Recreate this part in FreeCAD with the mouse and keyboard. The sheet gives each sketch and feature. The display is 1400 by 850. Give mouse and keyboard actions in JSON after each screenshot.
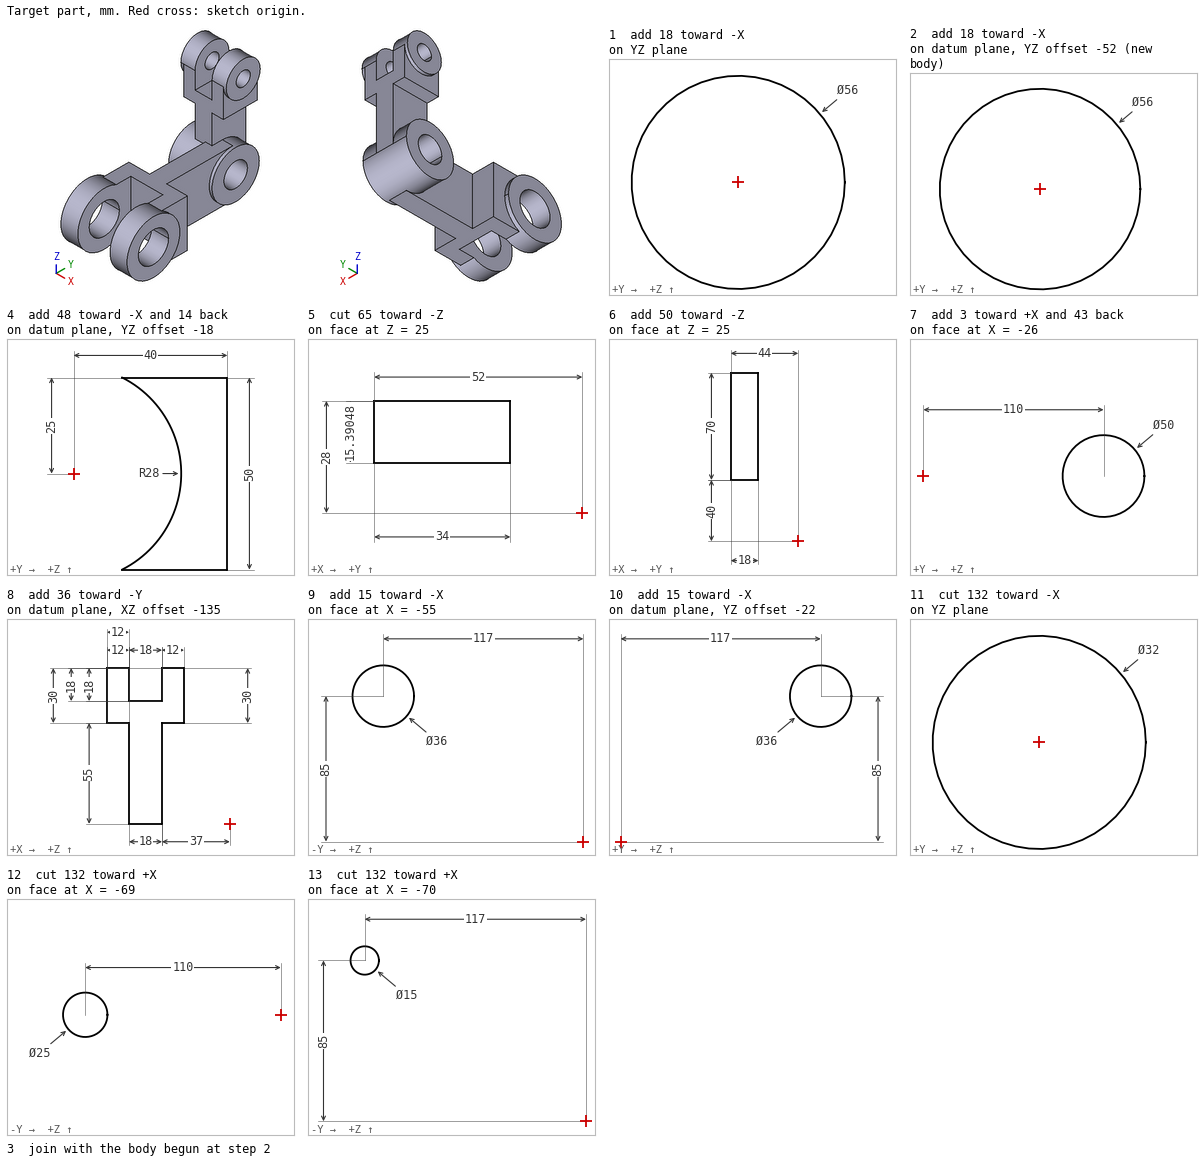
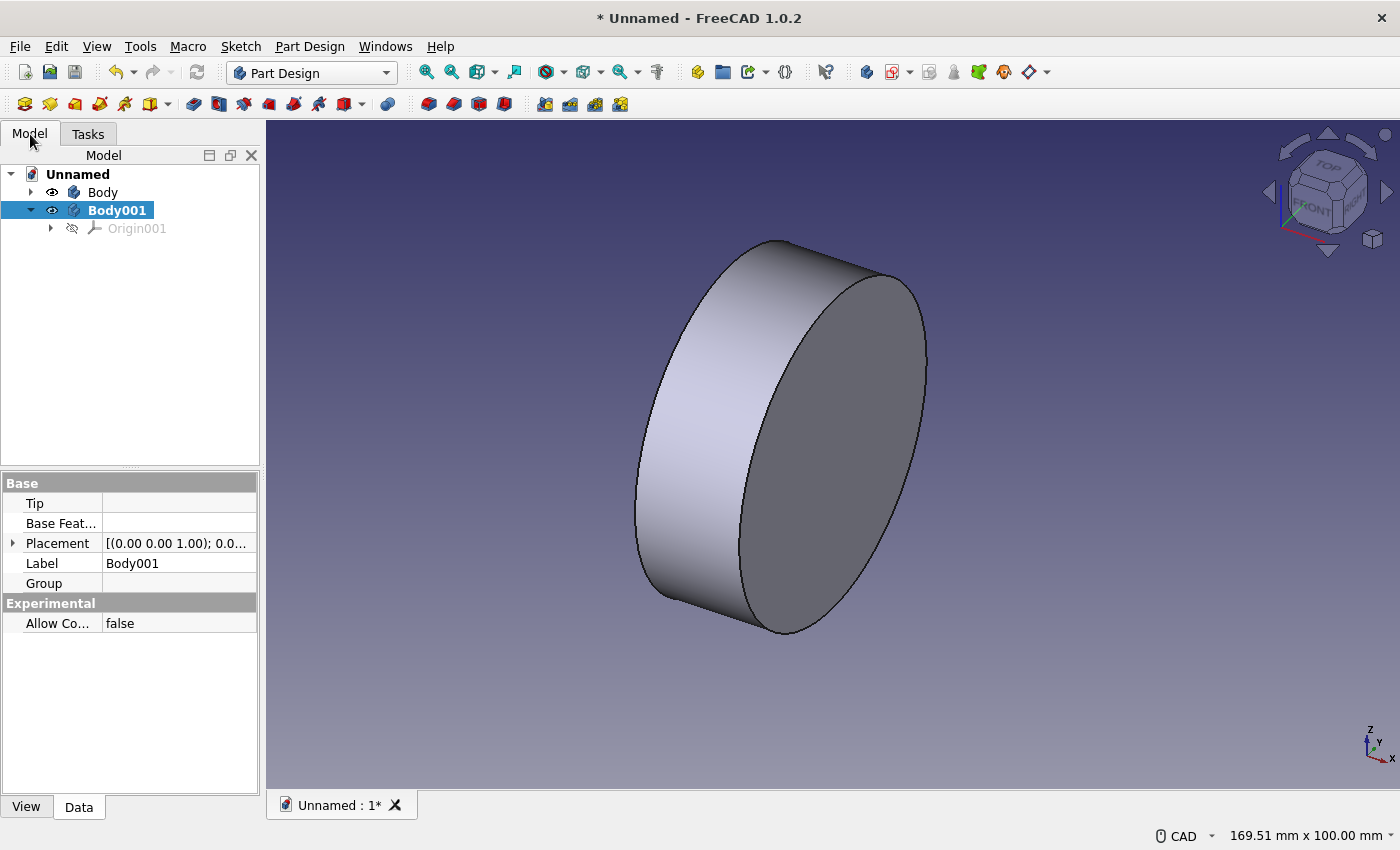
{"action": "left_click", "coordinate": [51, 228]}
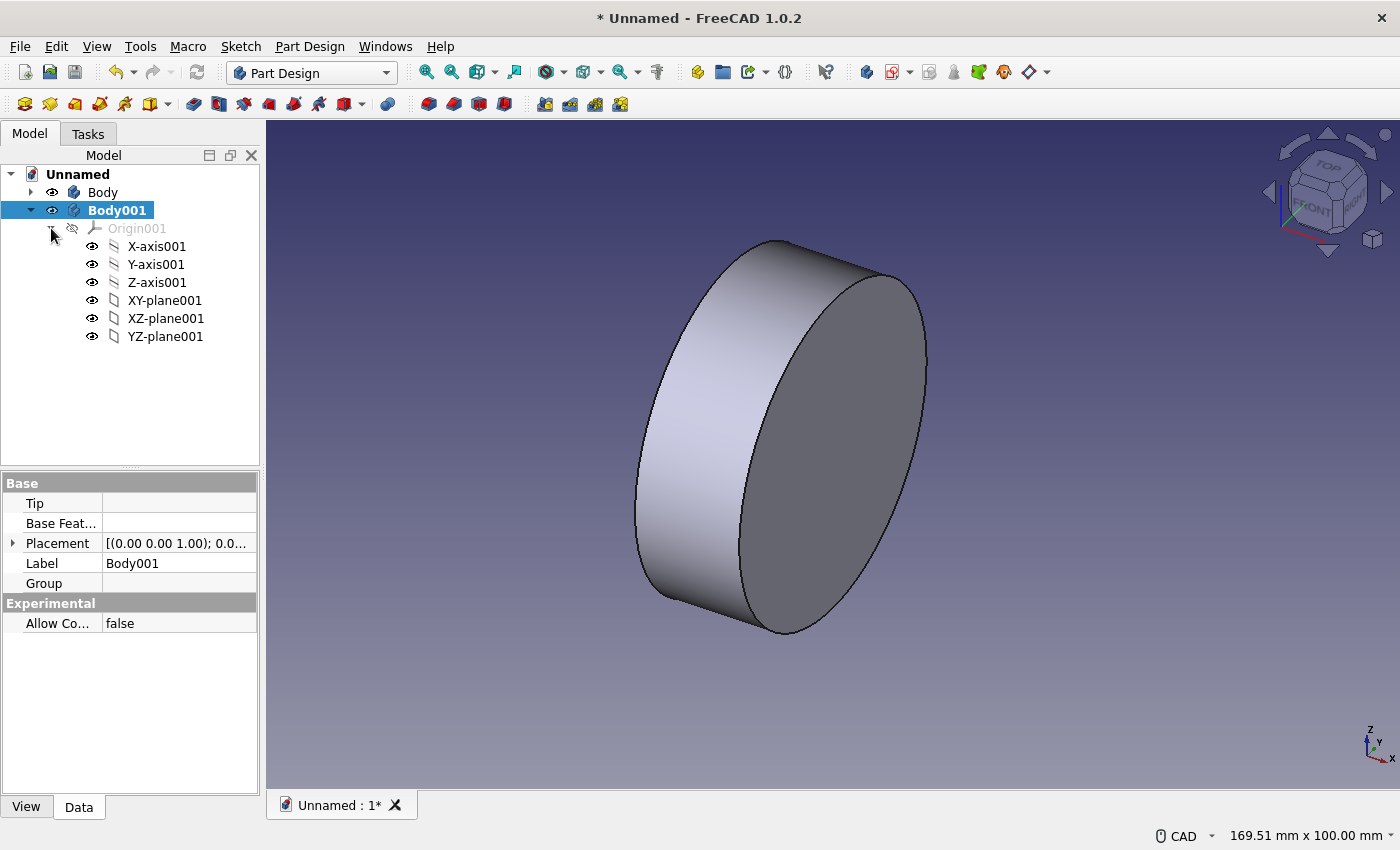
{"action": "left_click", "coordinate": [137, 336]}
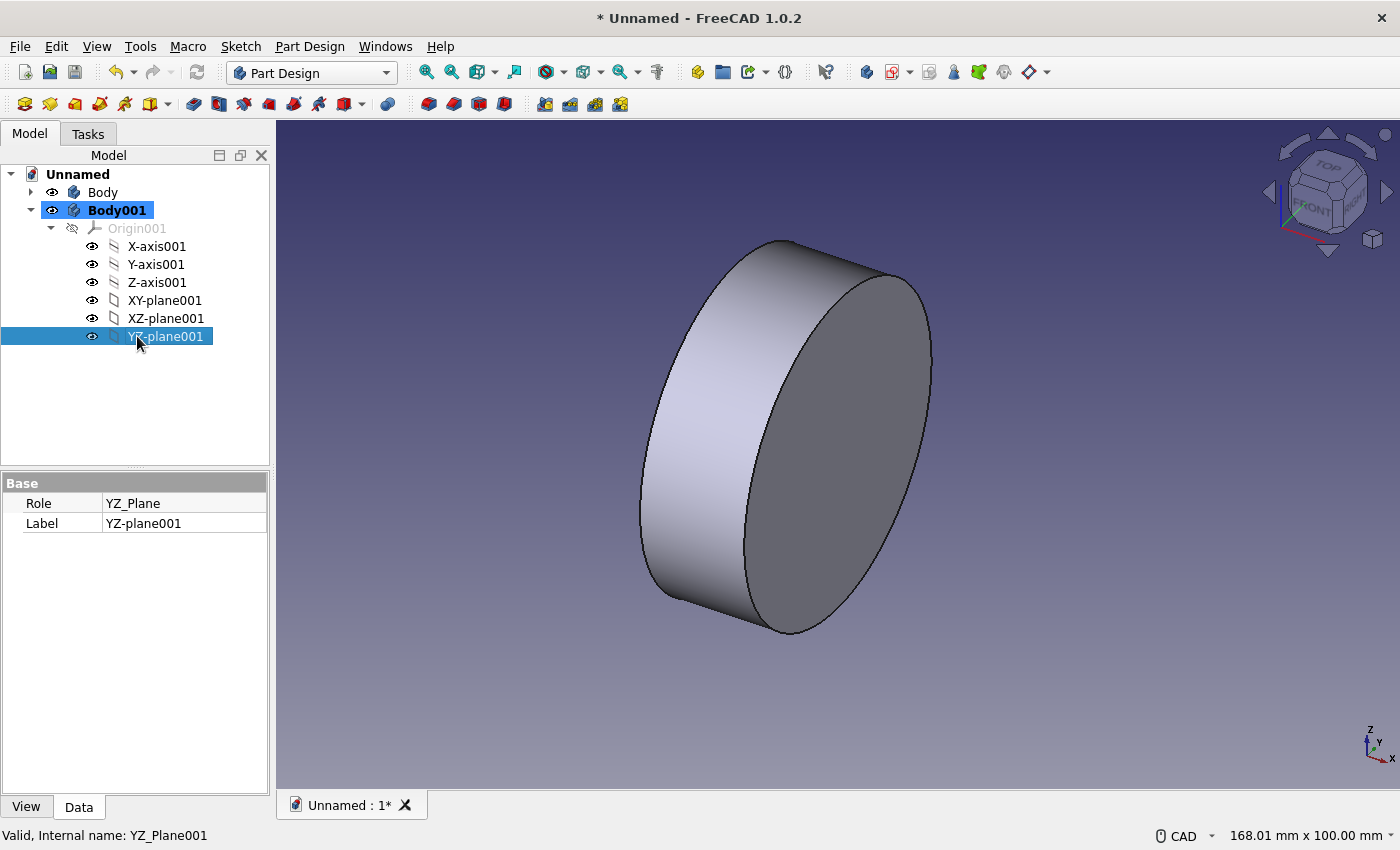
{"action": "left_click", "coordinate": [1028, 72]}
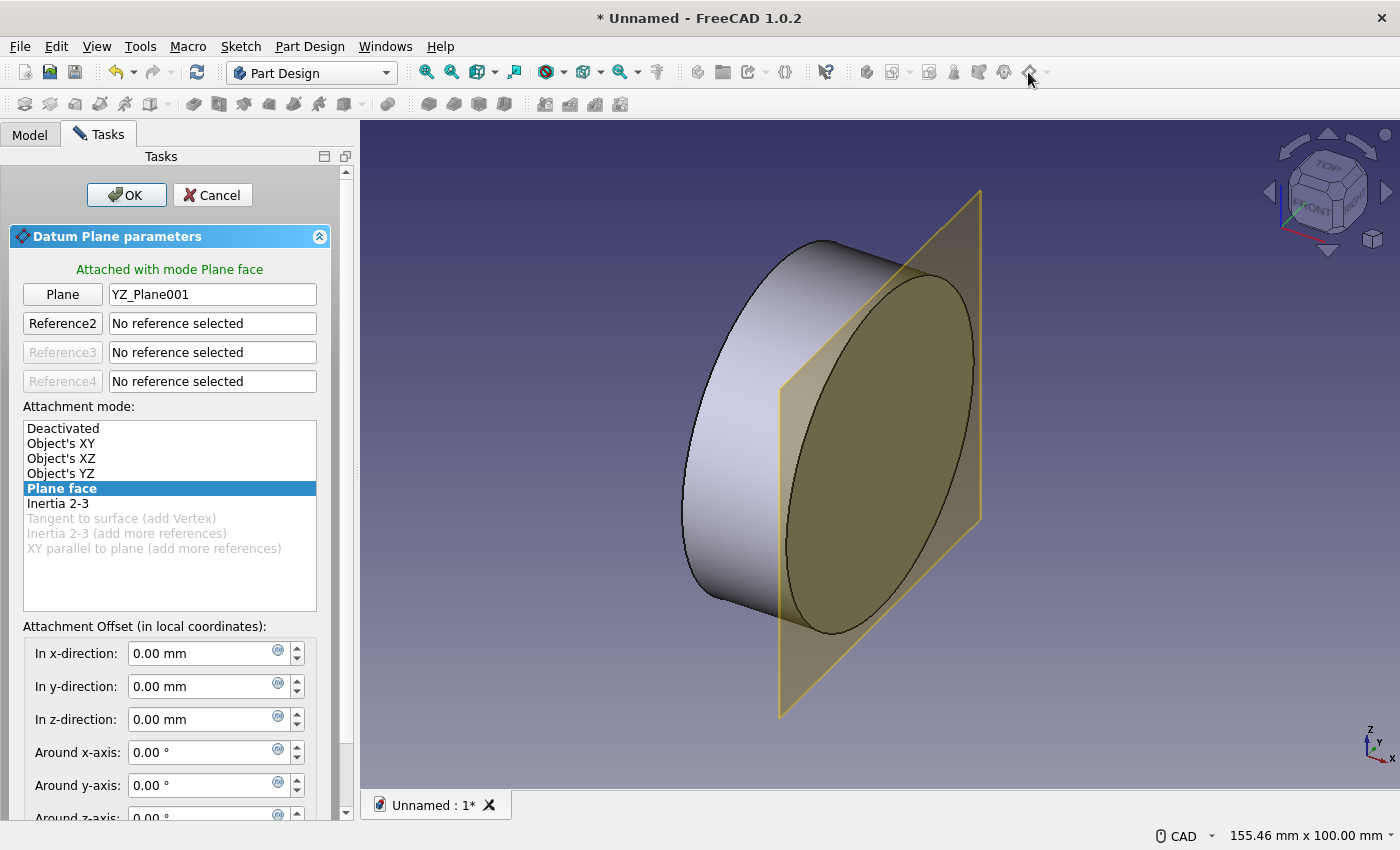
{"action": "triple_click", "coordinate": [210, 720]}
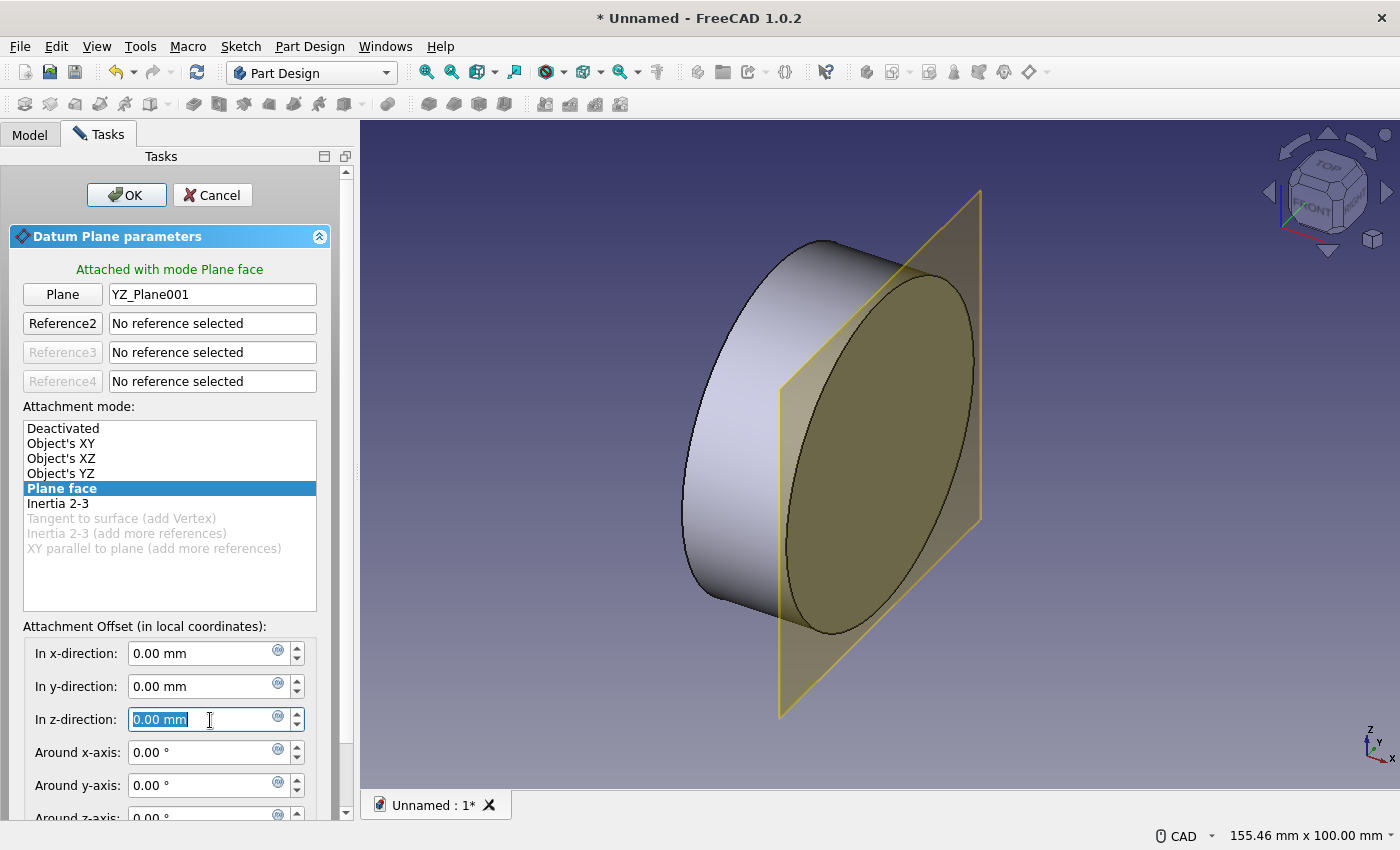
{"action": "type", "text": "-52"}
{"action": "key", "text": "Tab"}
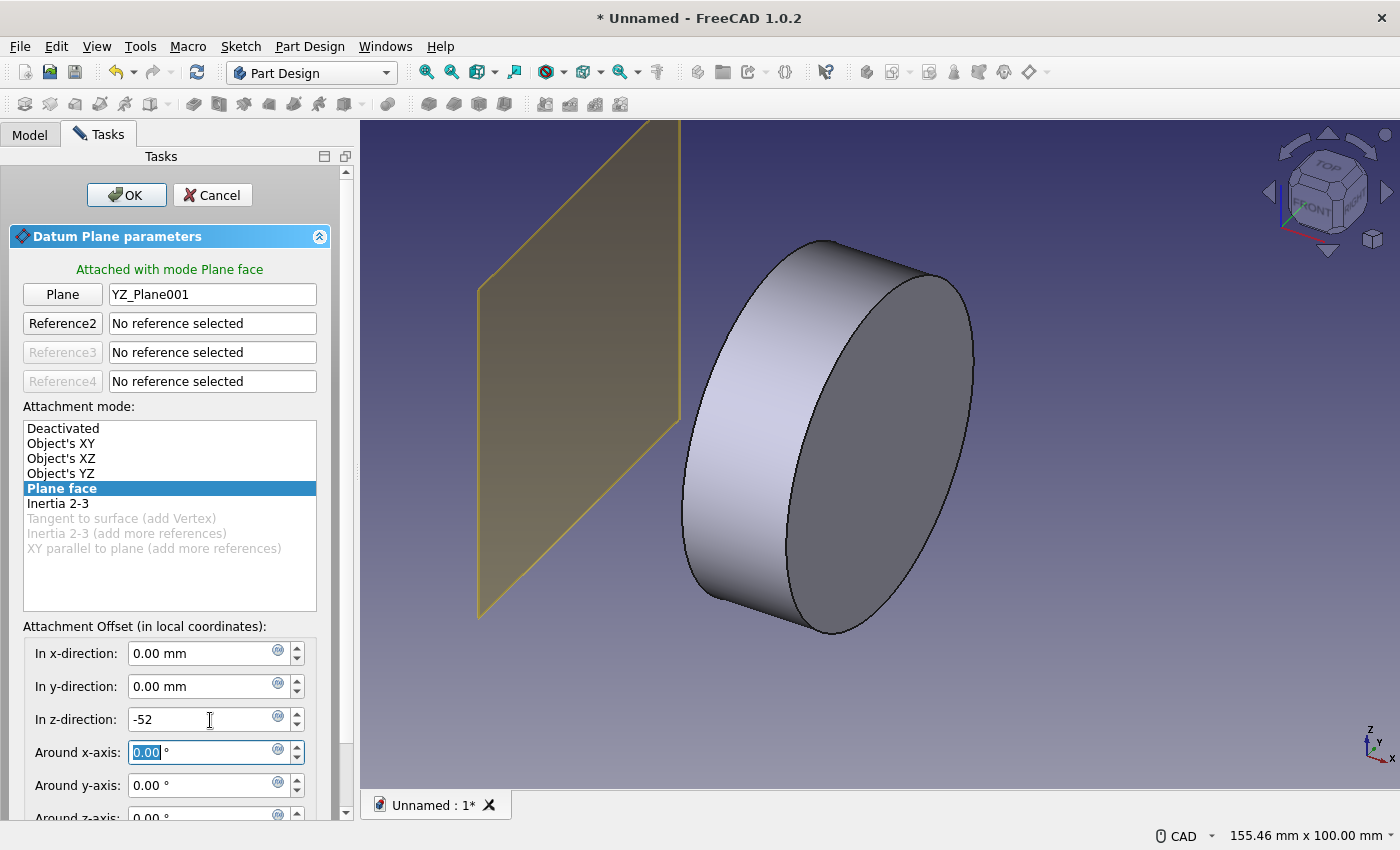
{"action": "left_click", "coordinate": [127, 195]}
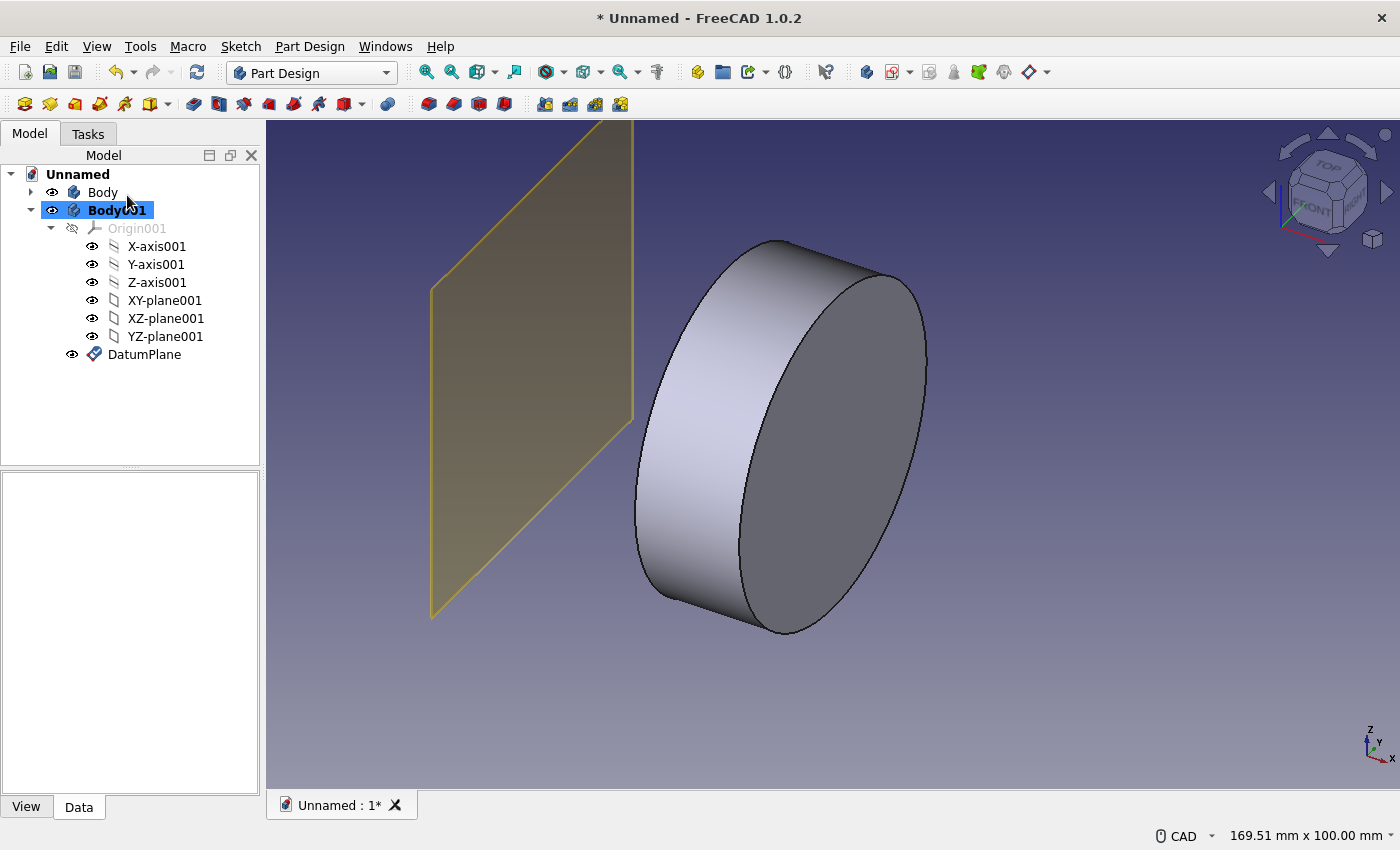
{"action": "left_click", "coordinate": [117, 354]}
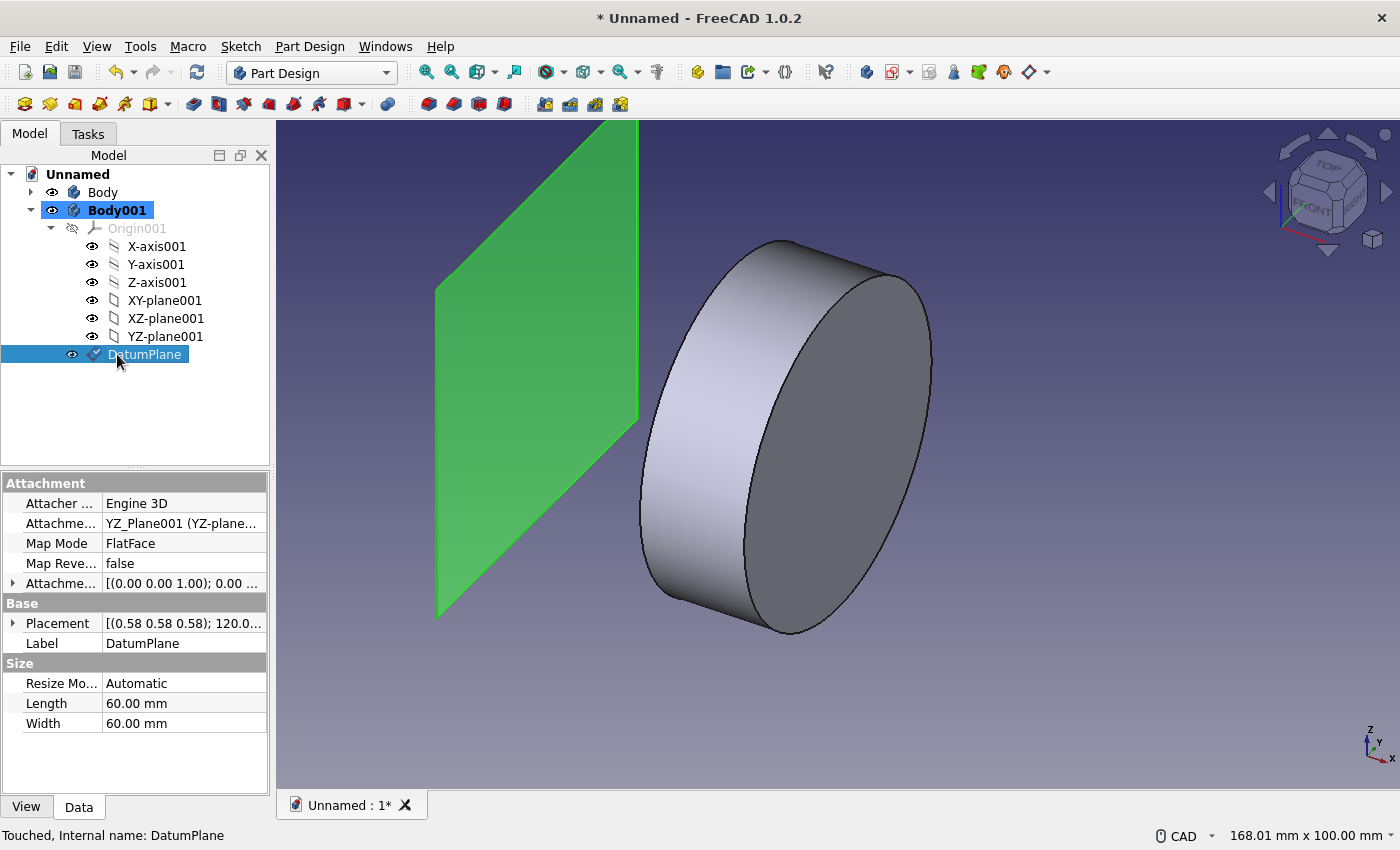
{"action": "left_click", "coordinate": [892, 72]}